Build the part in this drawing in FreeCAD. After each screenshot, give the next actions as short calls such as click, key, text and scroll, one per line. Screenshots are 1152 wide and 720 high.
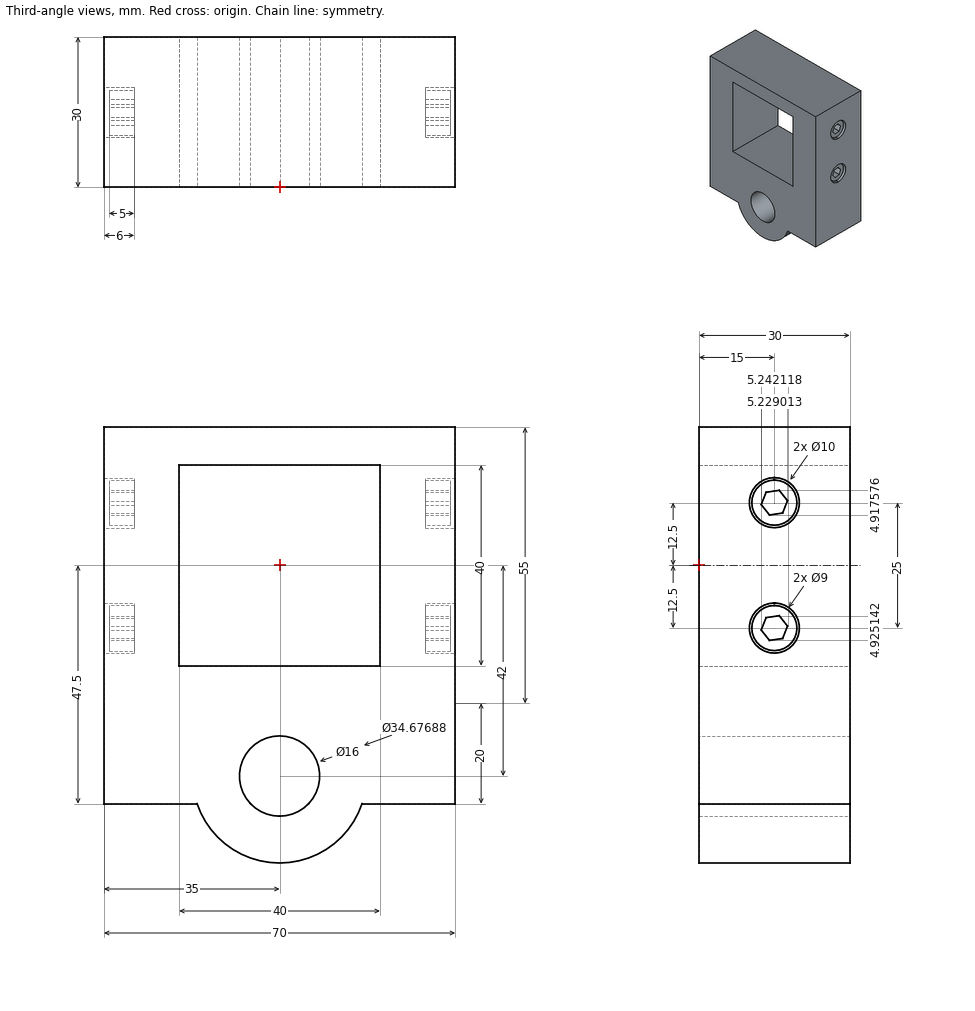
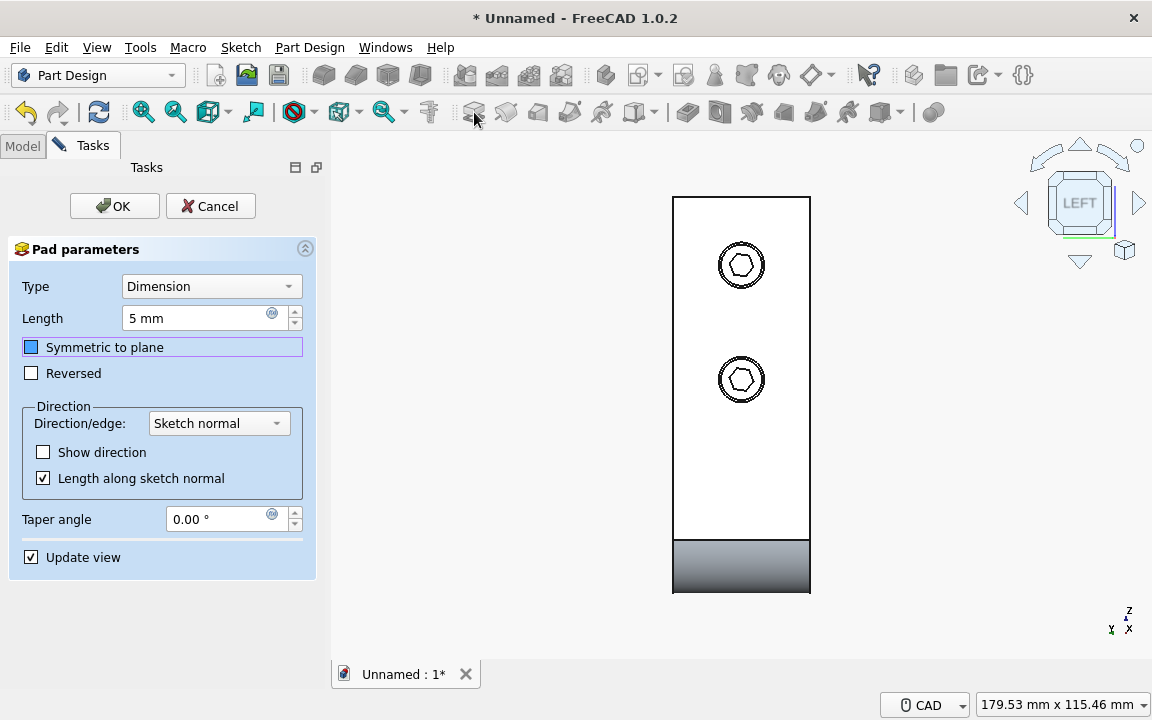
click(115, 206)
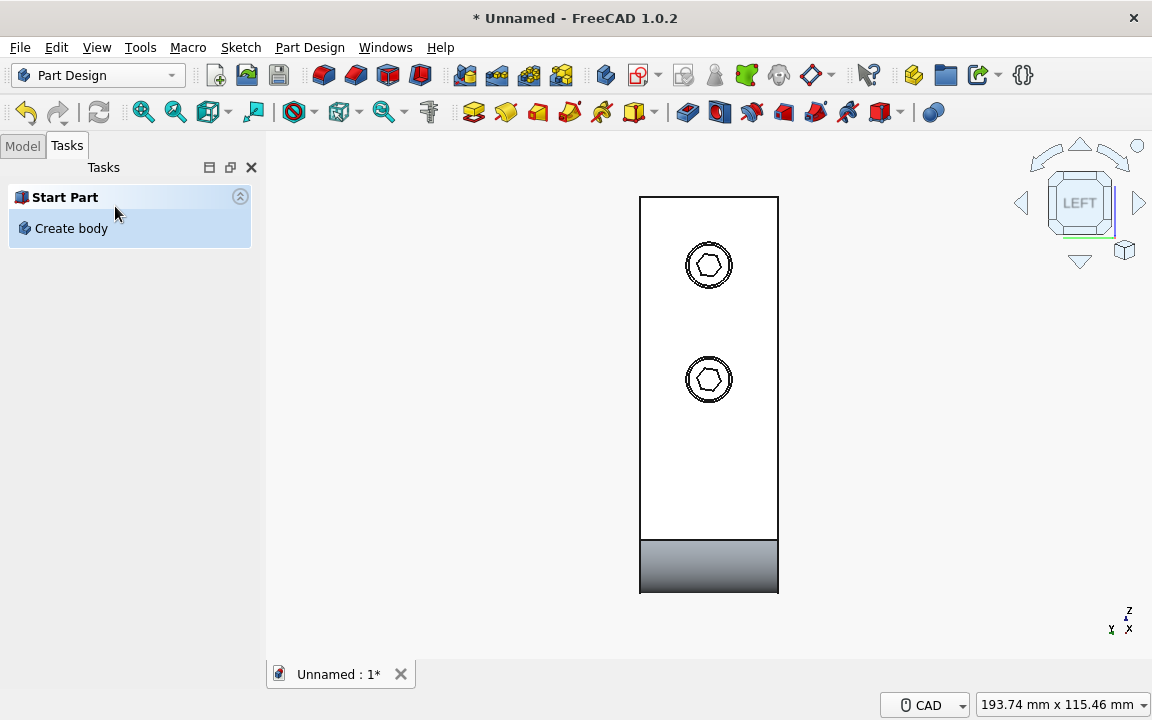
click(23, 145)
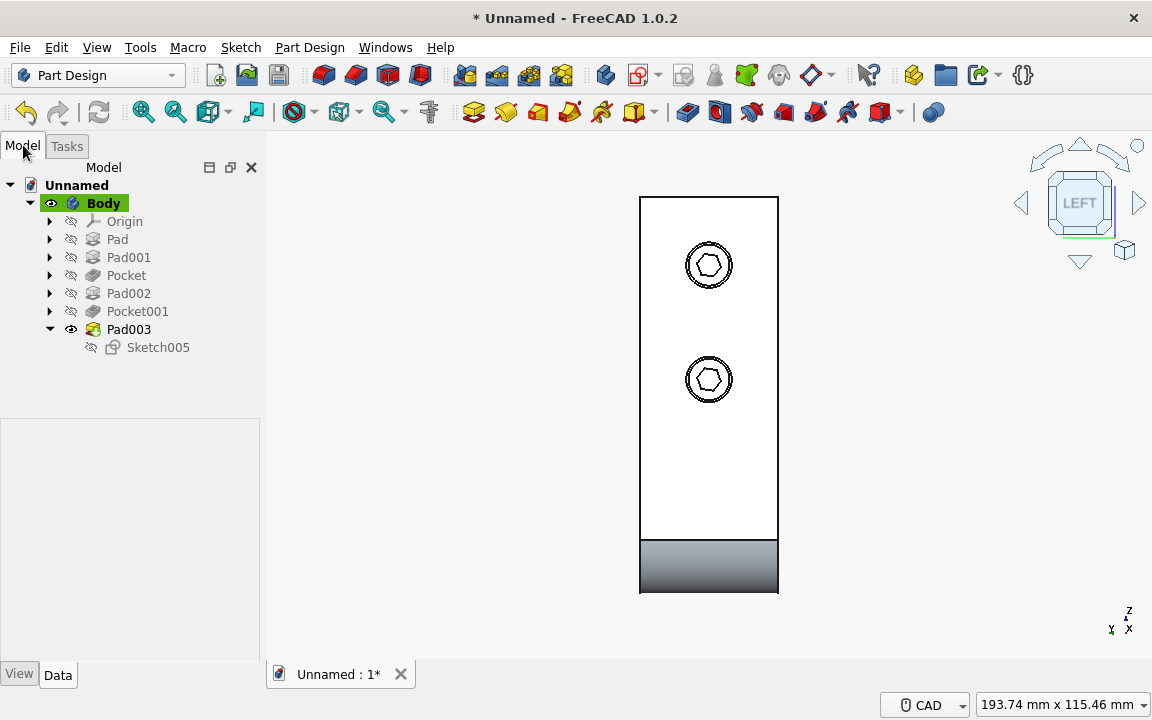
click(116, 311)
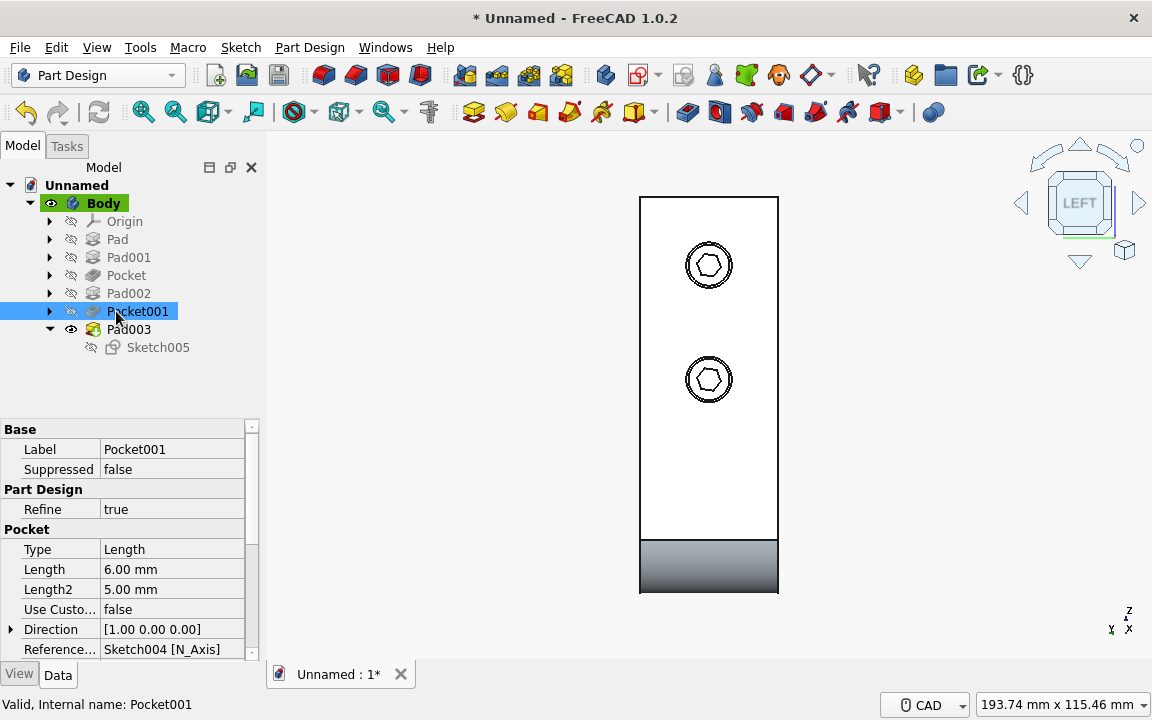
click(116, 329, ctrl)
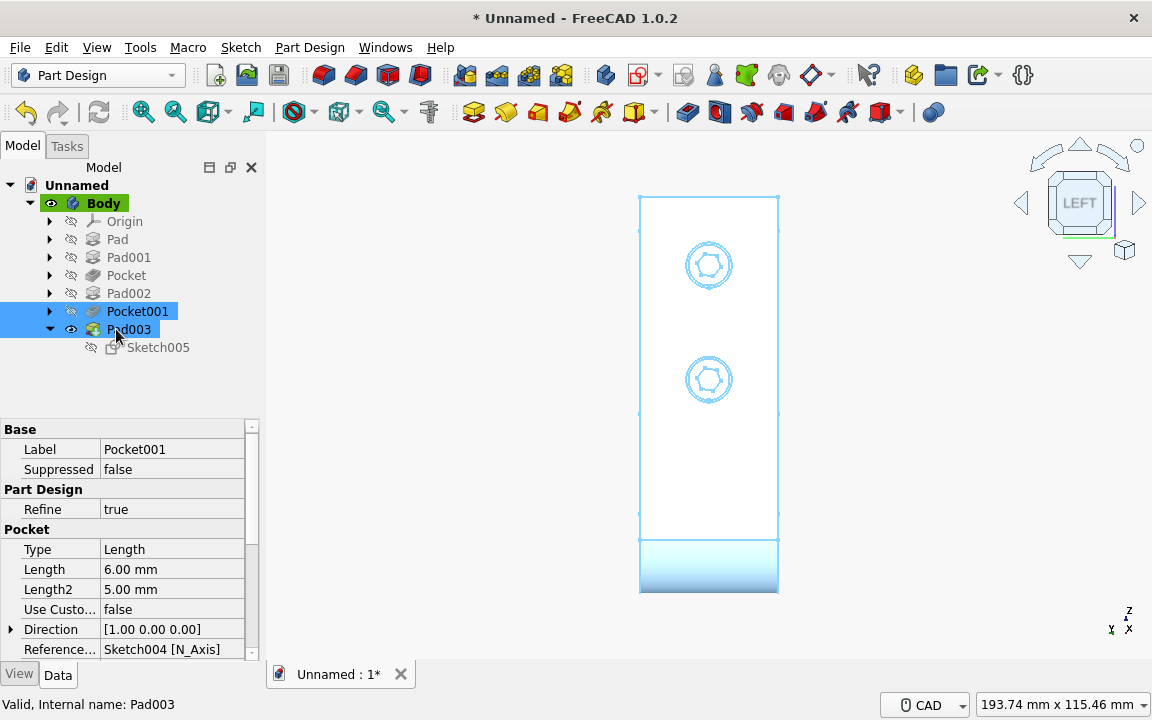
click(466, 76)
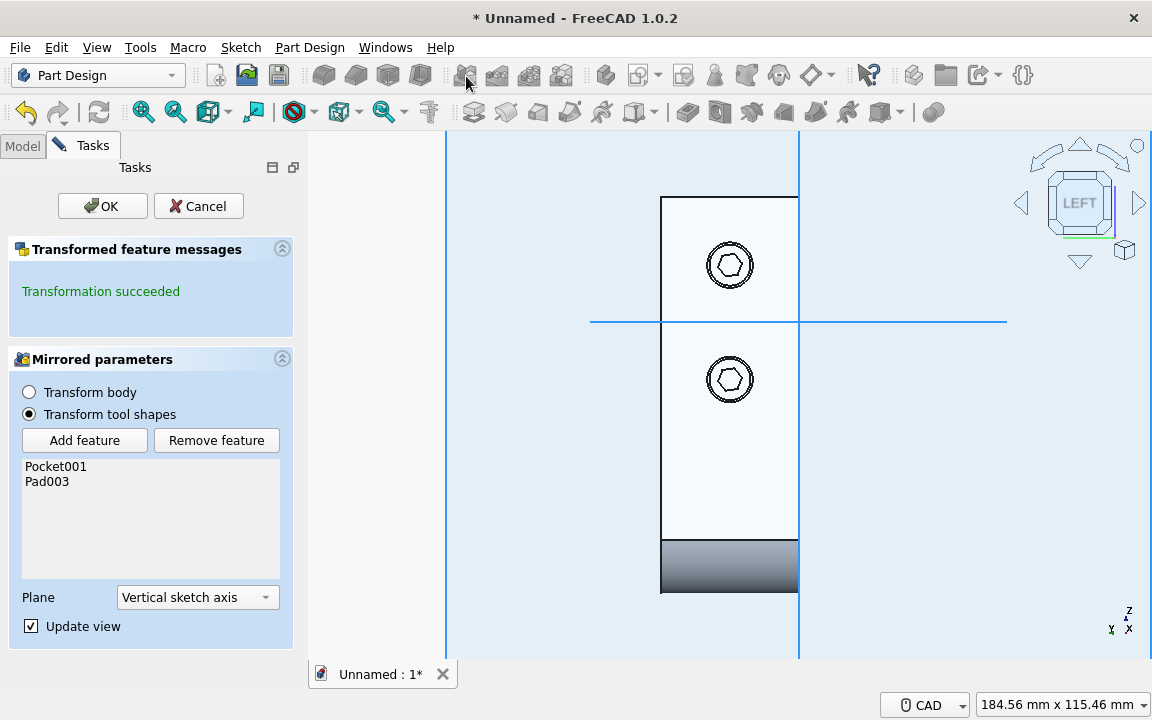
click(198, 598)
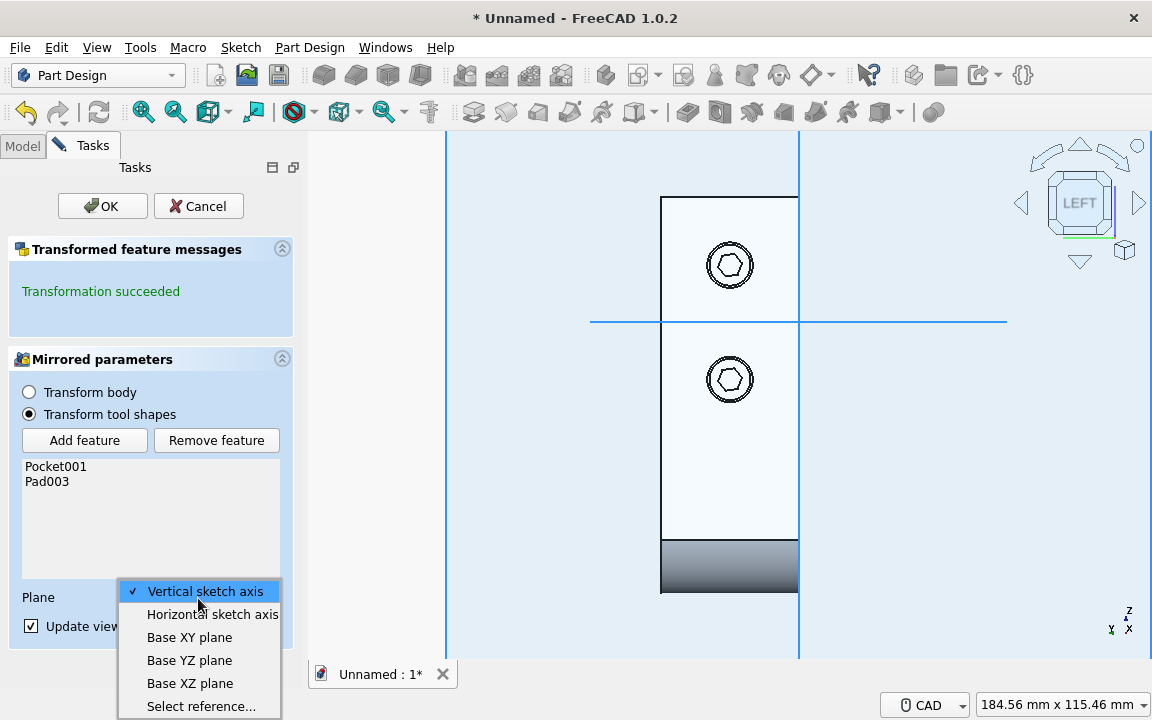
click(198, 660)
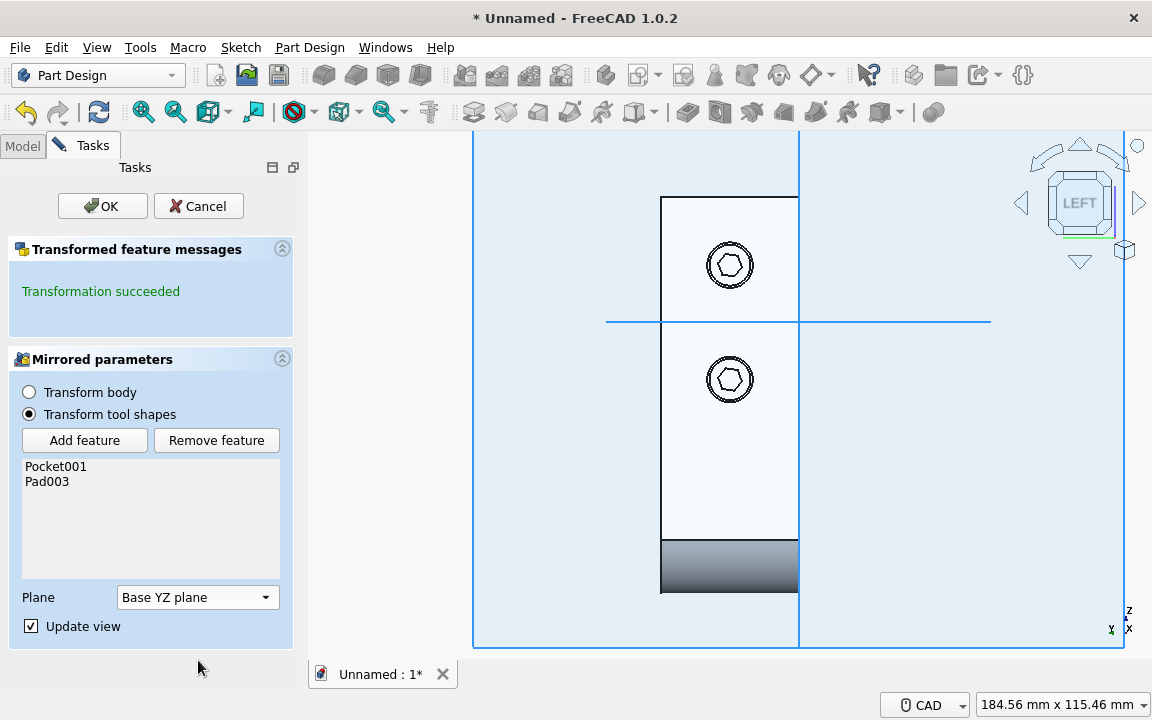
click(103, 206)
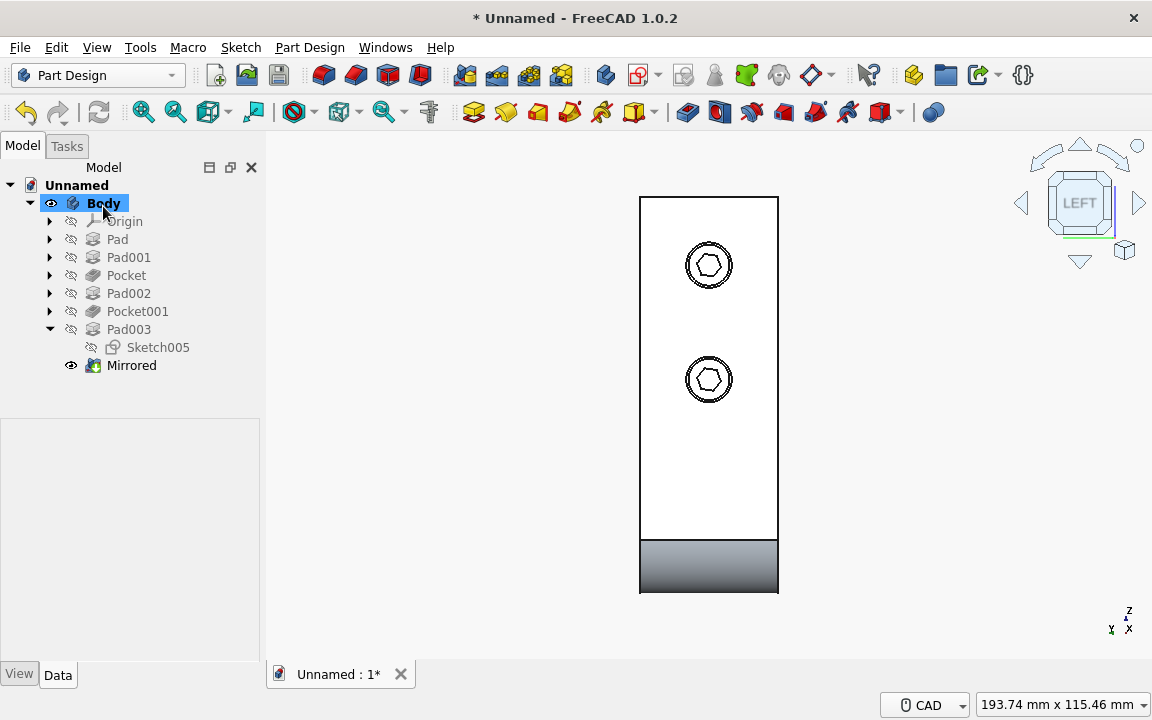
key(0)